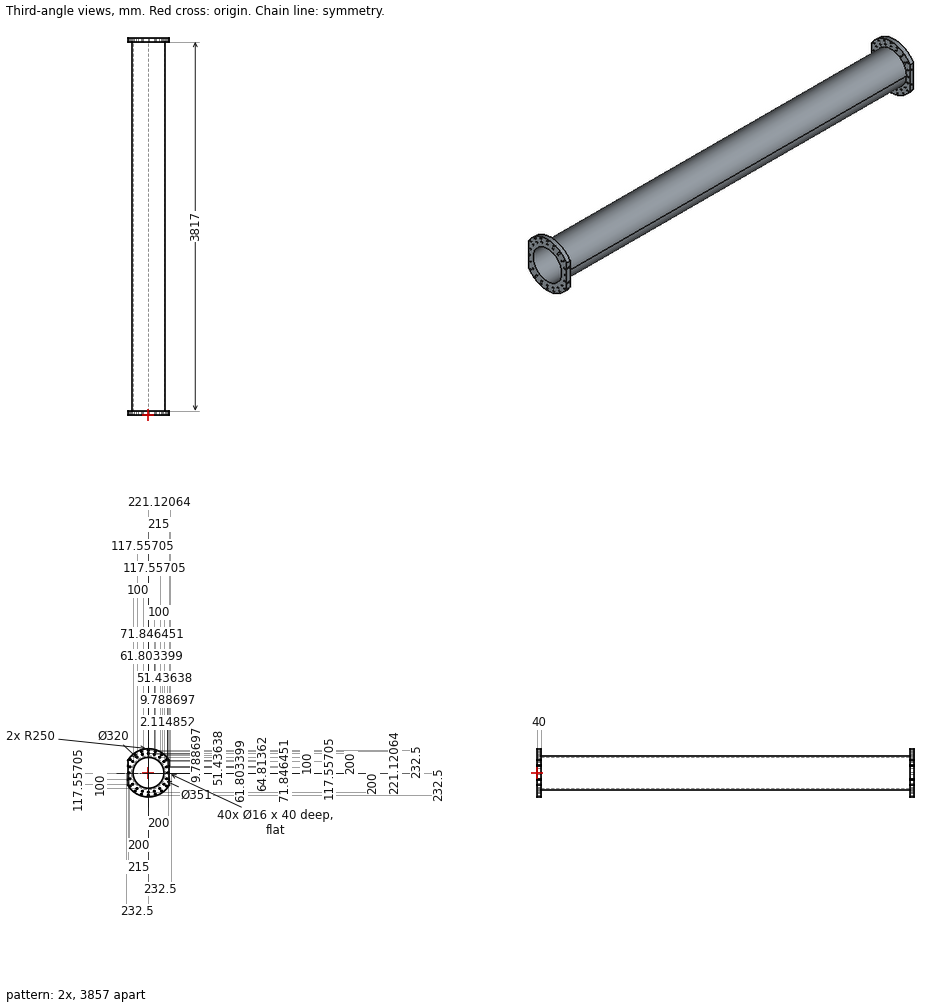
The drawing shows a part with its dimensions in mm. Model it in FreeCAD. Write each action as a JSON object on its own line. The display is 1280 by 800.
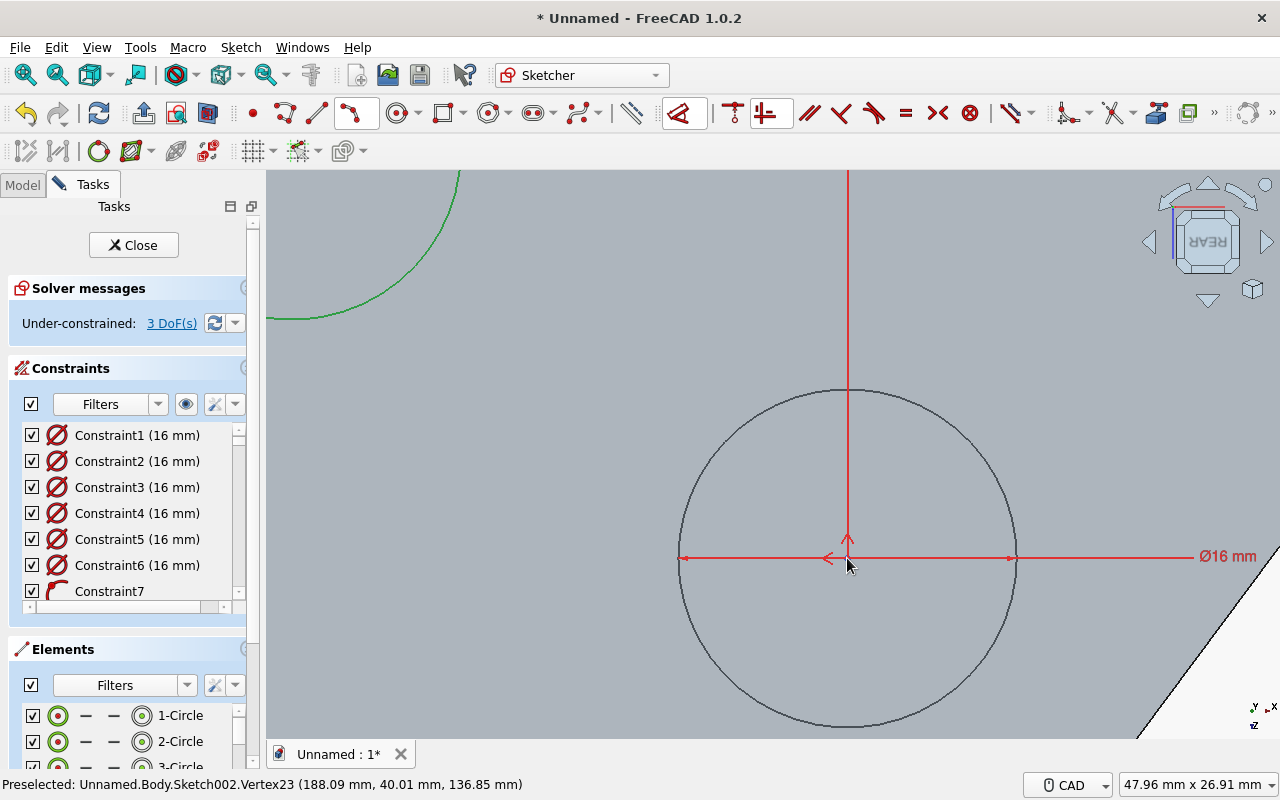
{"action": "scroll", "coordinate": [867, 573], "scroll_direction": "down", "scroll_amount": 16}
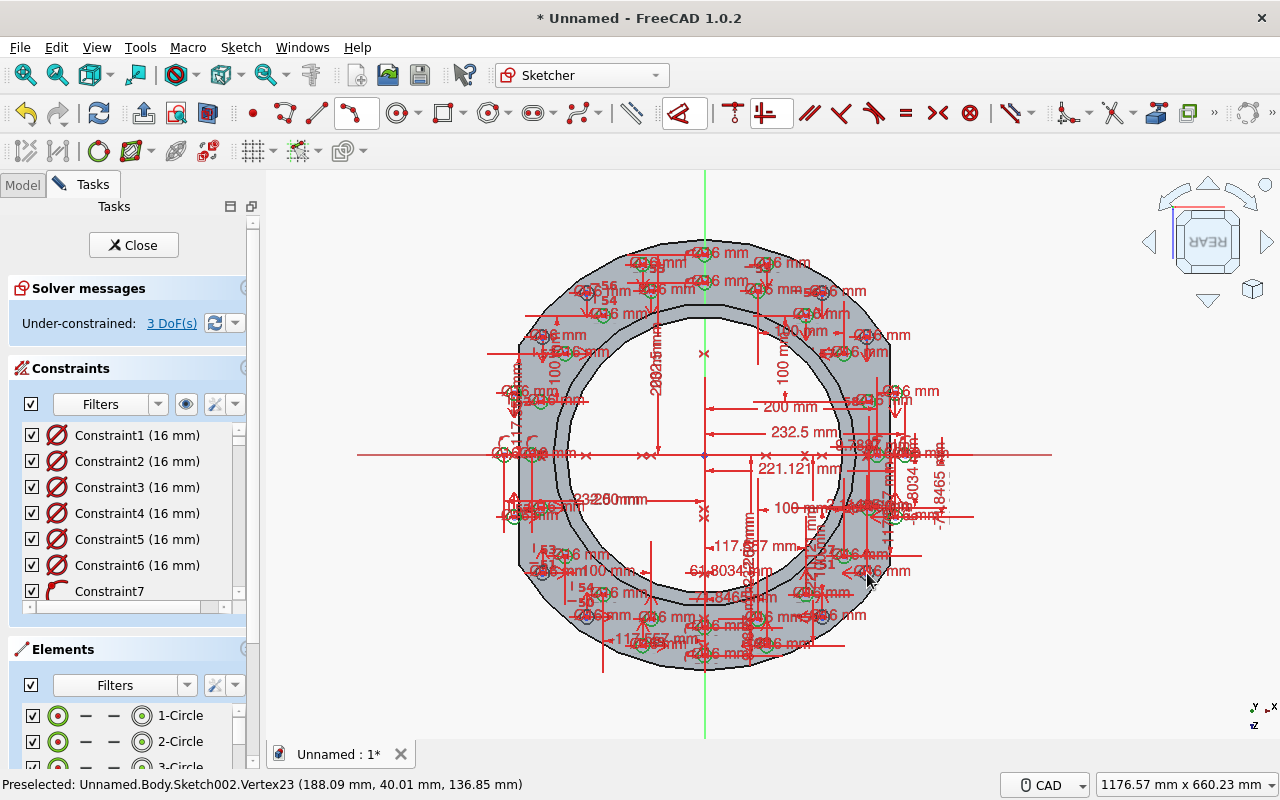
{"action": "left_click", "coordinate": [895, 517]}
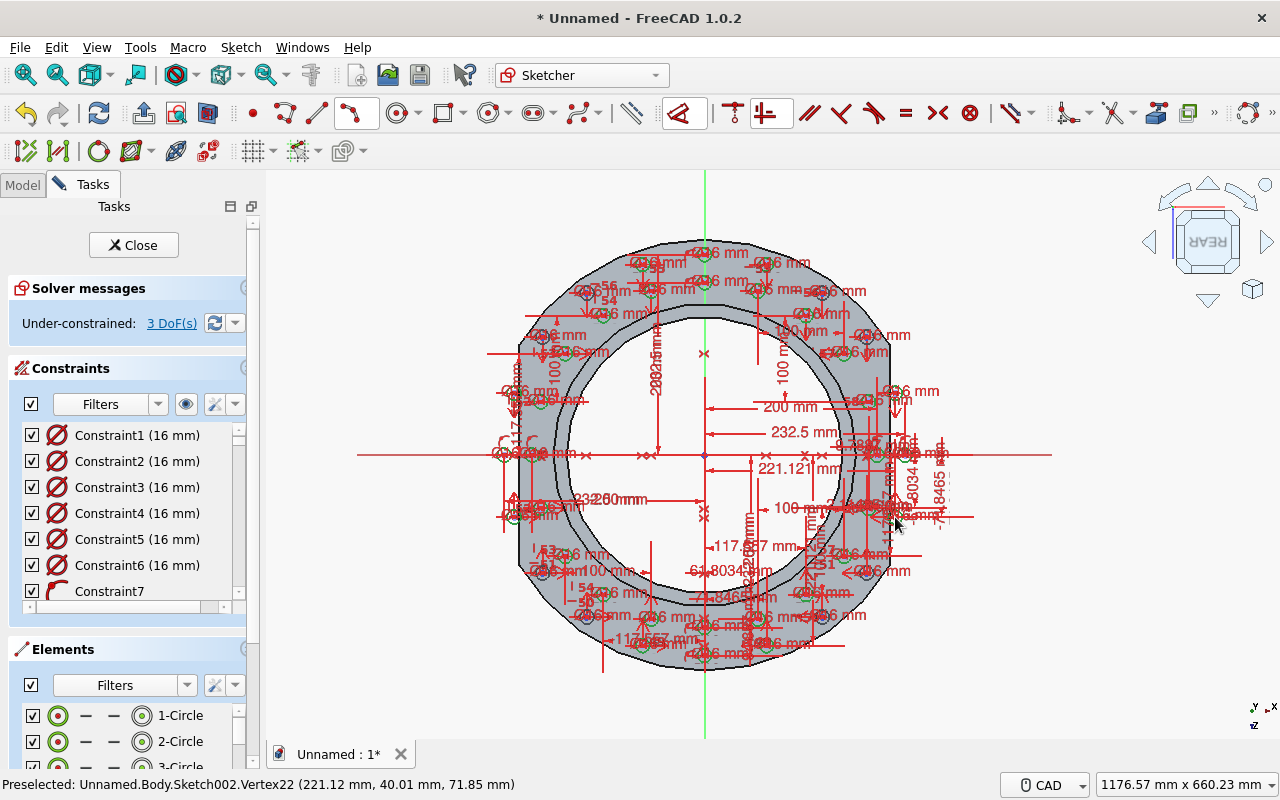
{"action": "left_click", "coordinate": [867, 573]}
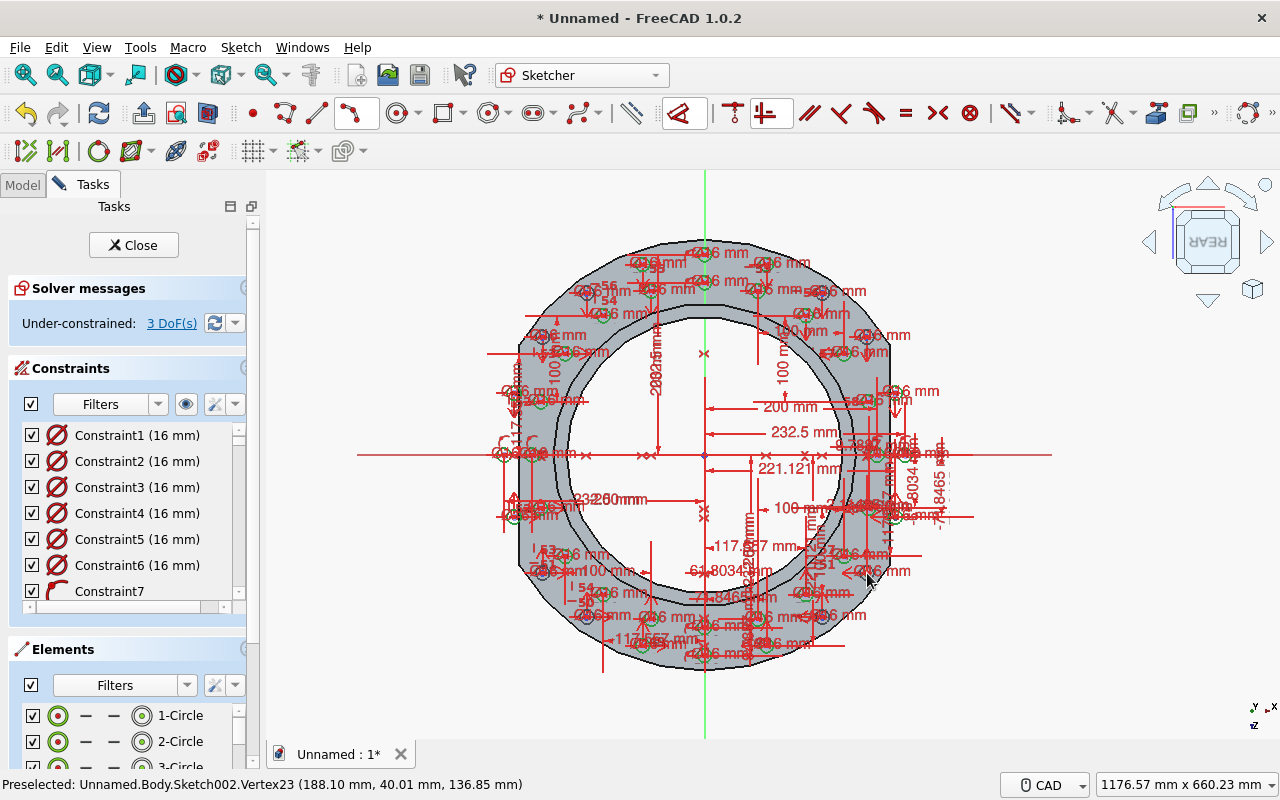
{"action": "left_click", "coordinate": [702, 114]}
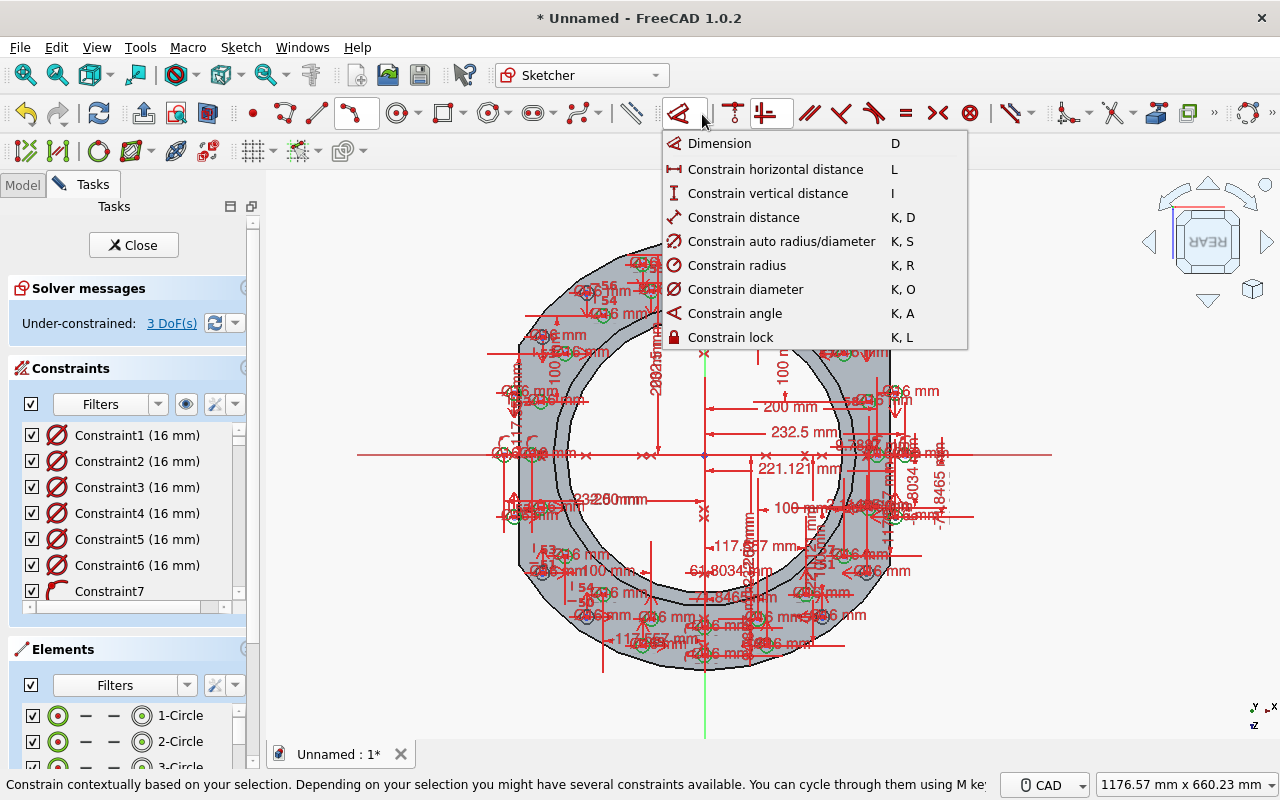
{"action": "left_click", "coordinate": [815, 193]}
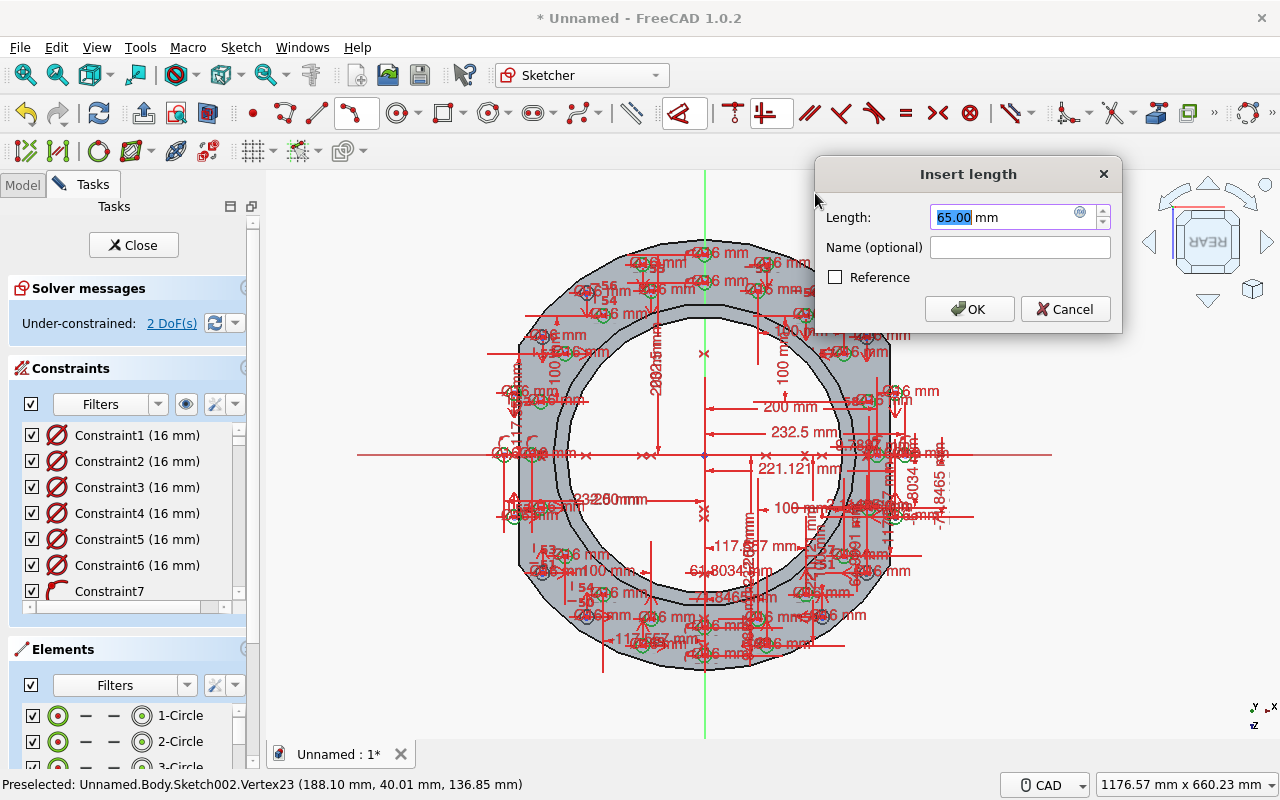
{"action": "type", "text": "64.81362"}
{"action": "key", "text": "Return"}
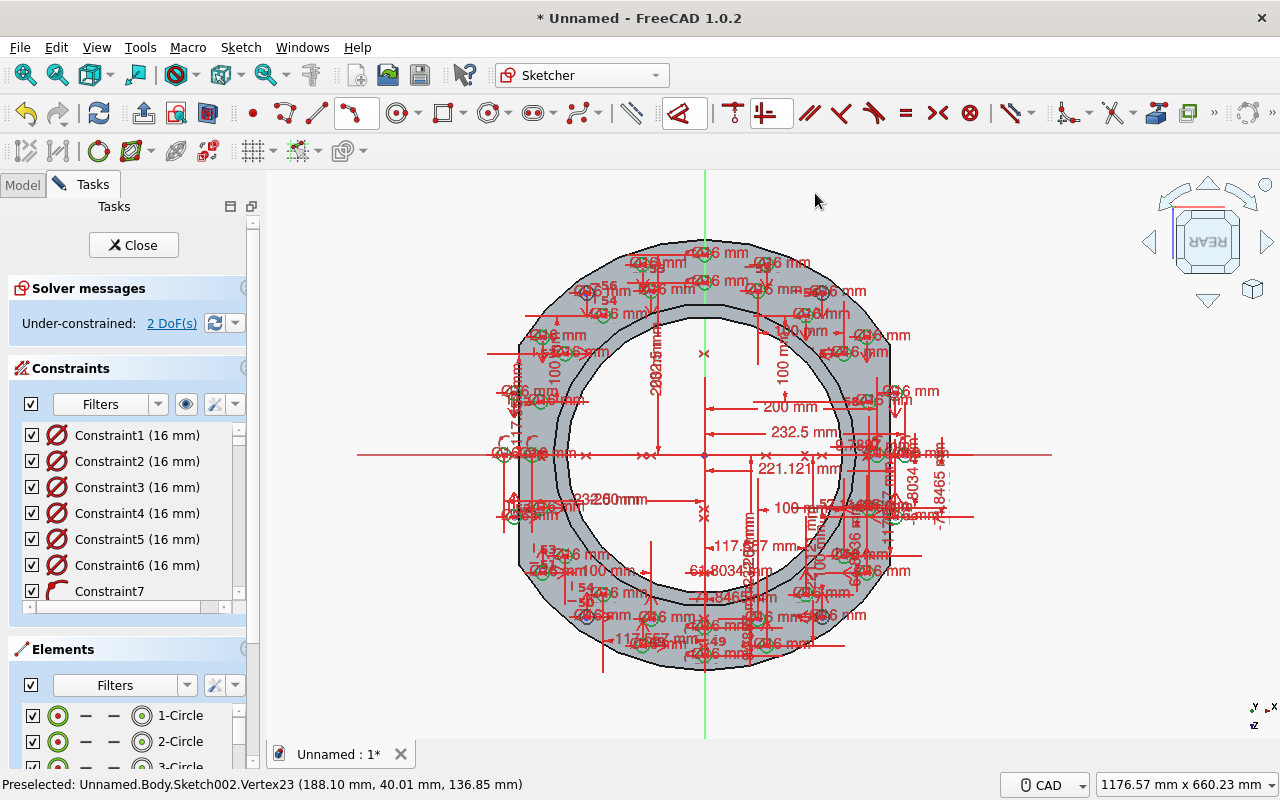
{"action": "left_click", "coordinate": [867, 573]}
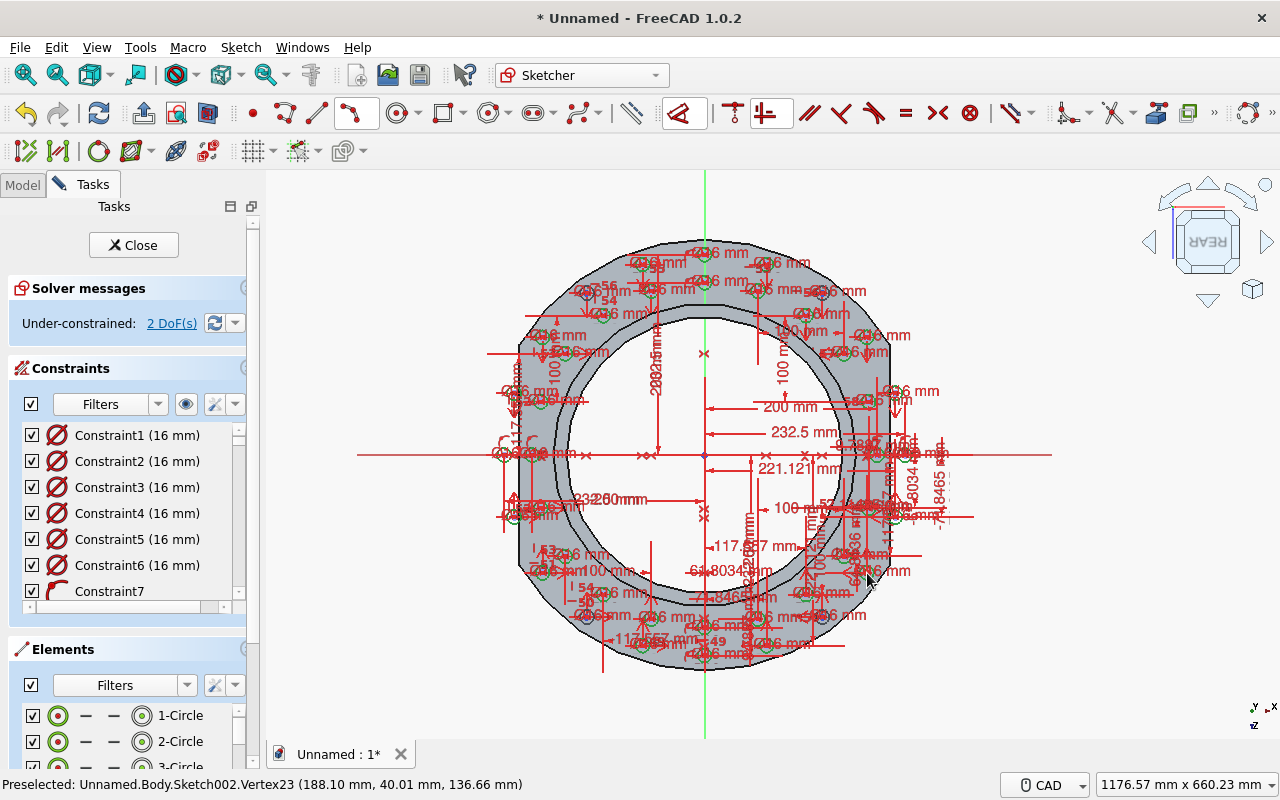
{"action": "left_click", "coordinate": [822, 617]}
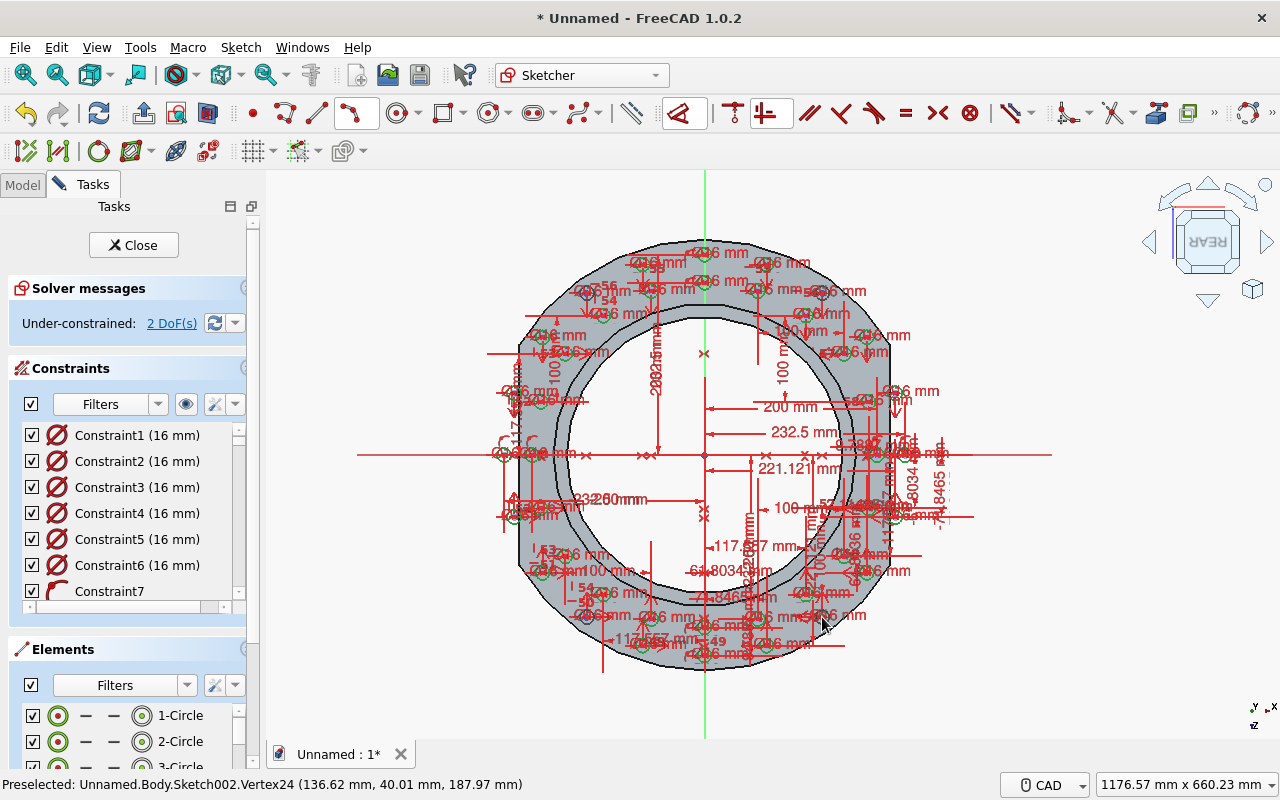
{"action": "left_click", "coordinate": [702, 114]}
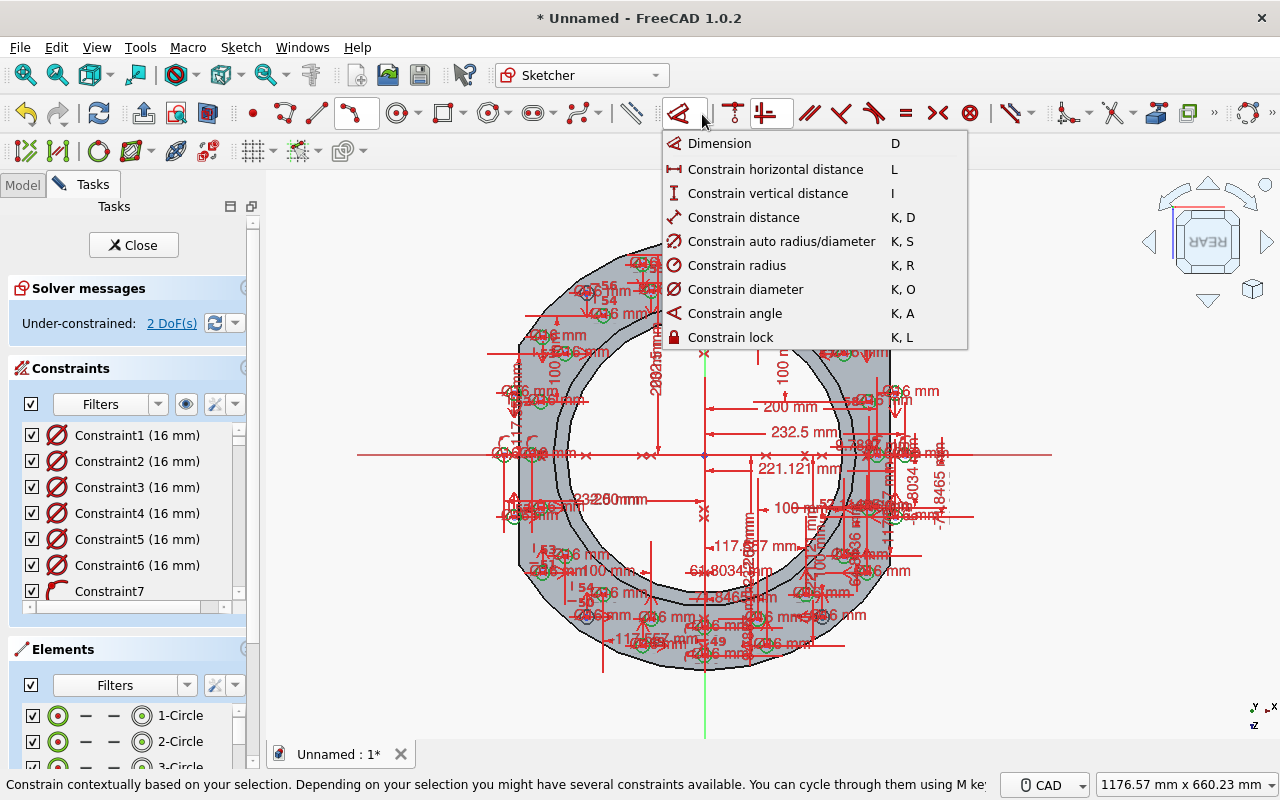
{"action": "left_click", "coordinate": [815, 169]}